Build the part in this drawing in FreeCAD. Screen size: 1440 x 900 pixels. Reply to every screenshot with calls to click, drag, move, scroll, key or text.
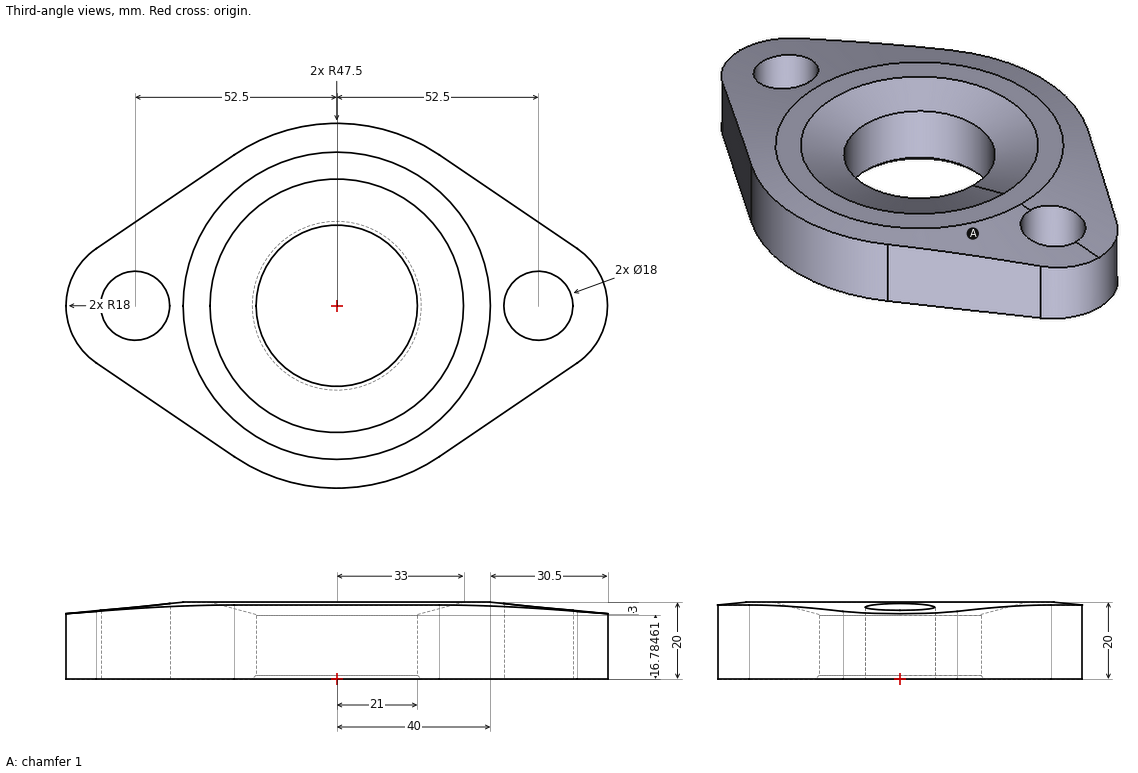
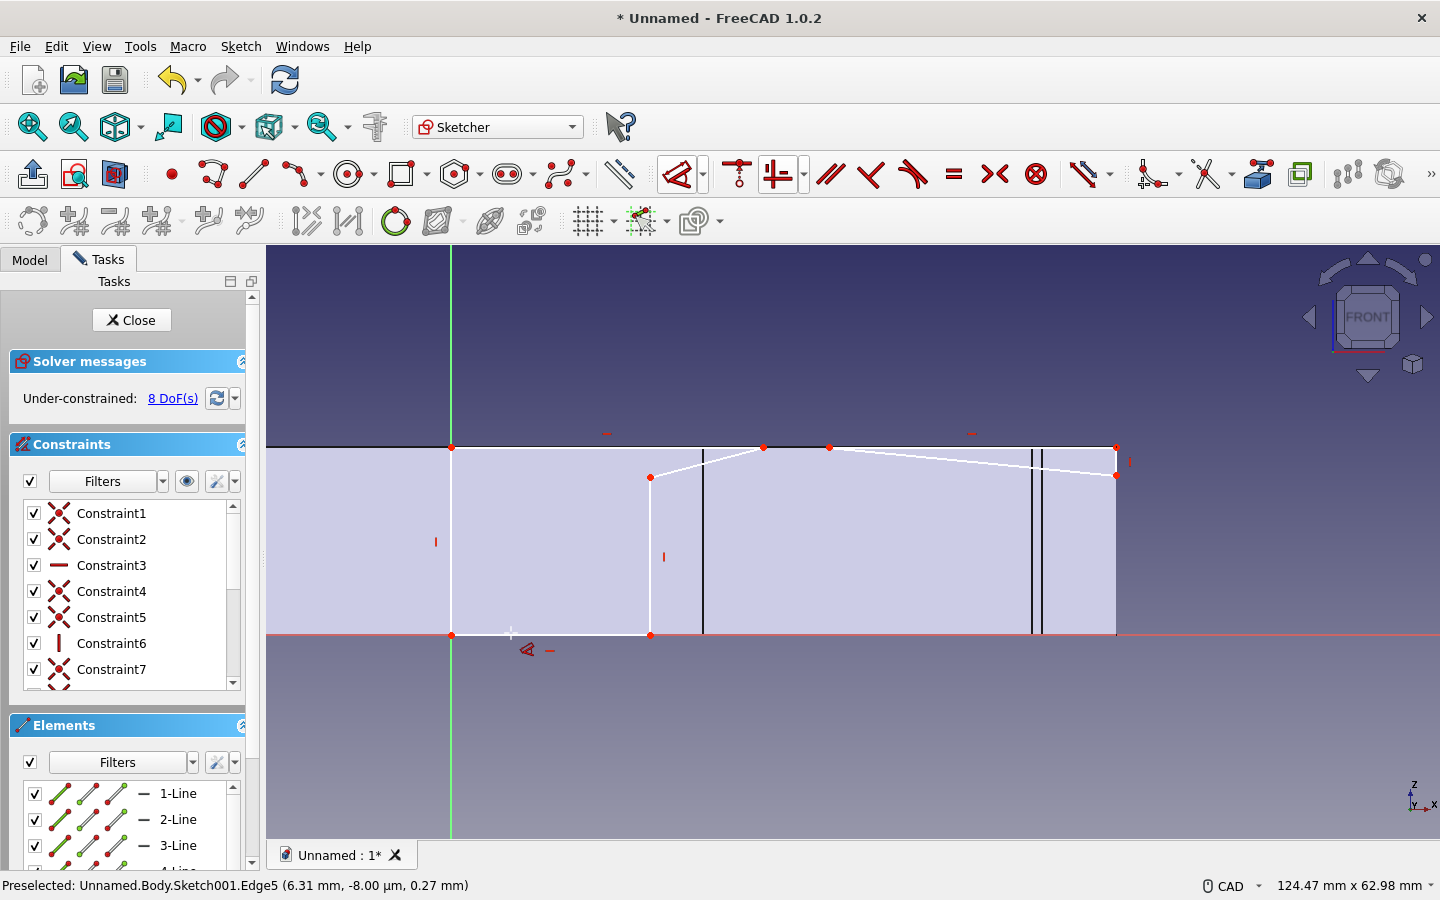
scroll(1116, 459, up, 2)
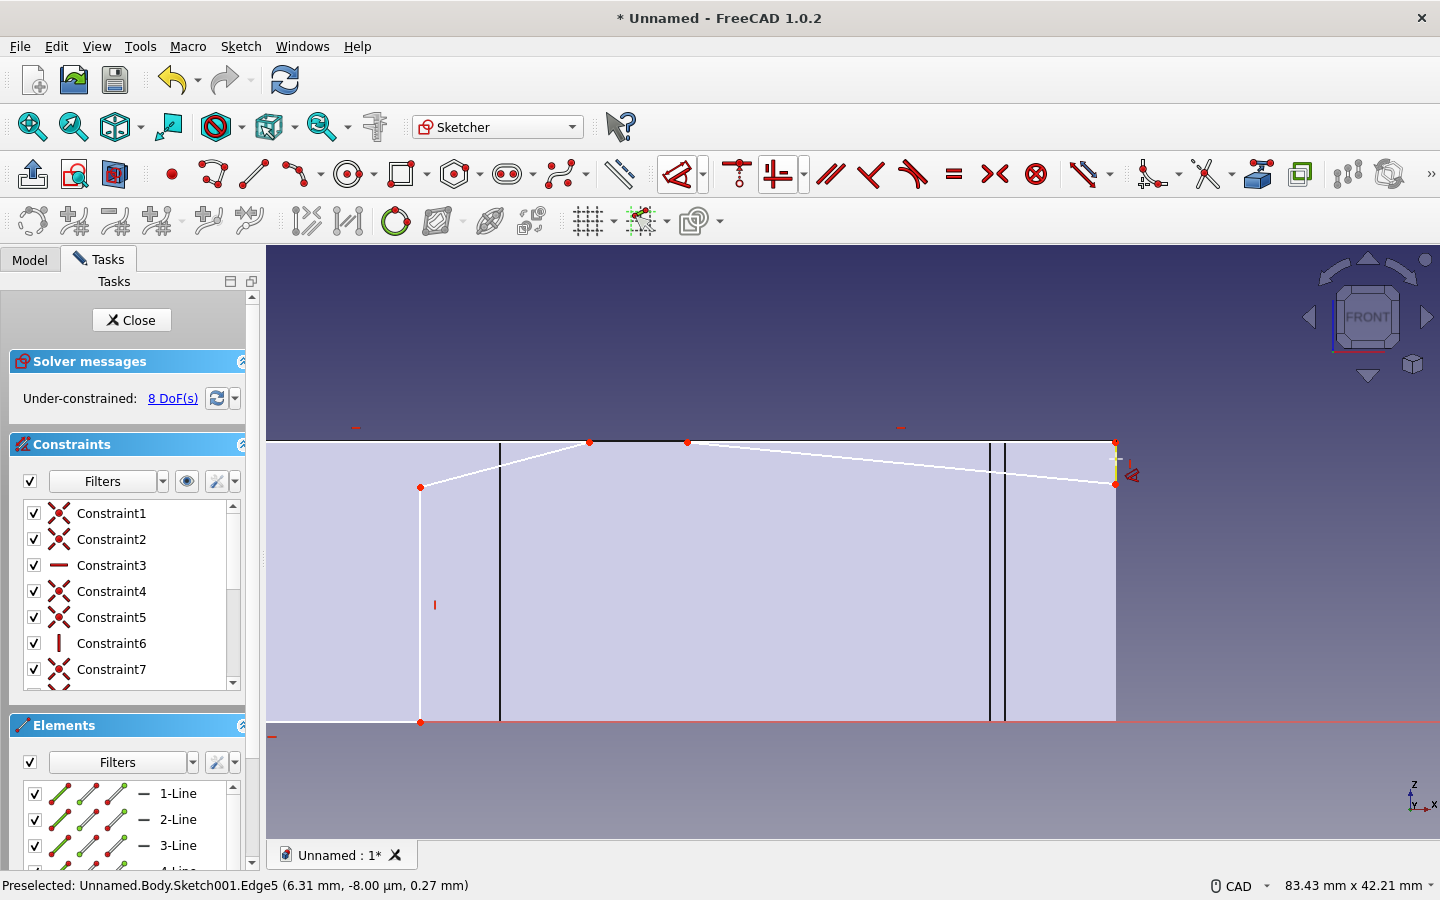
click(1116, 459)
click(1150, 463)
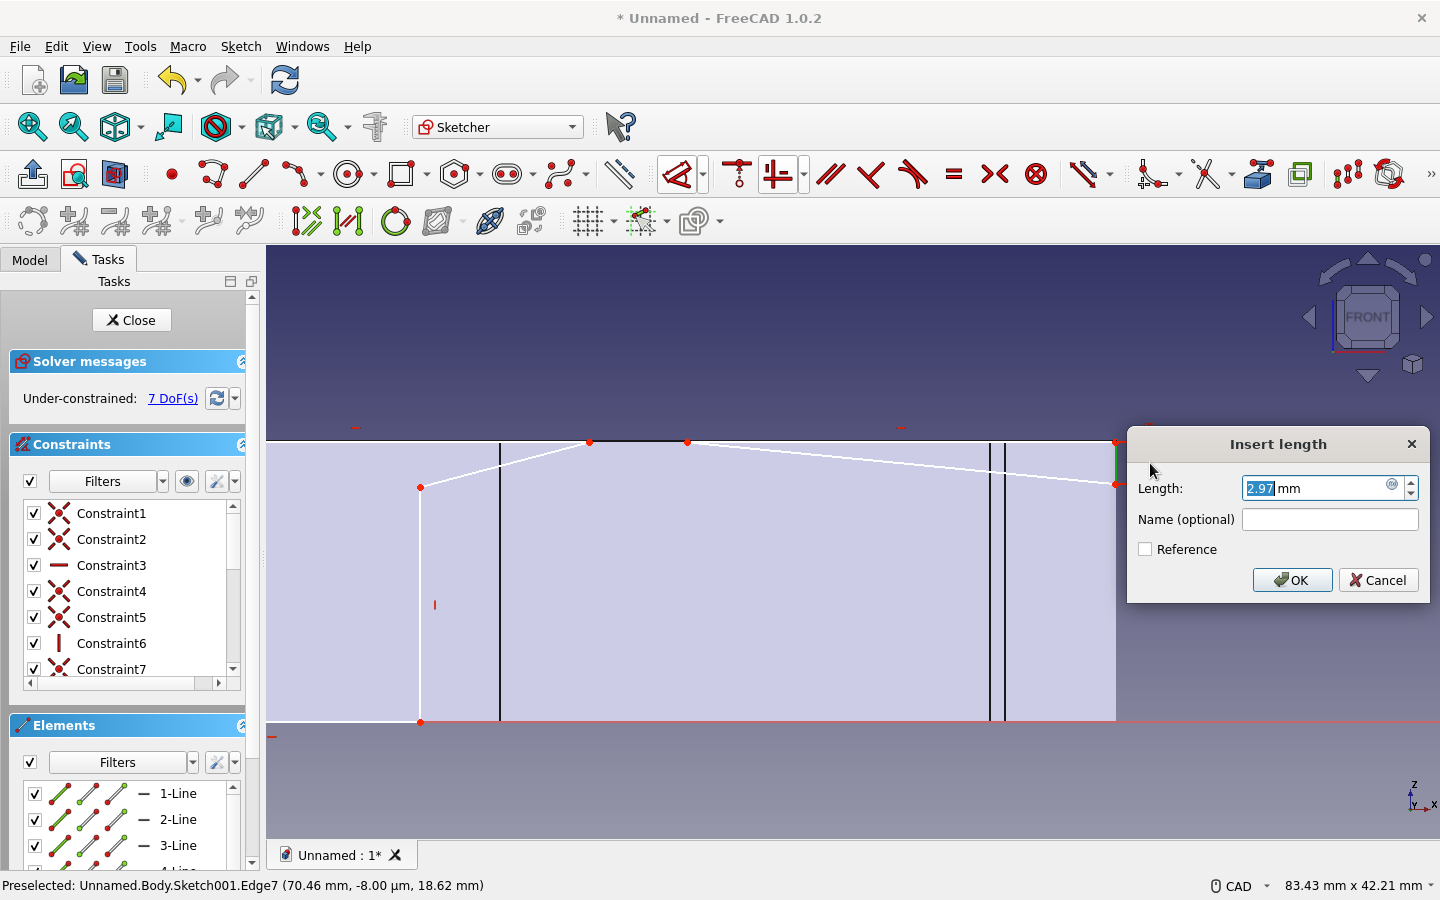
text(3)
key(Return)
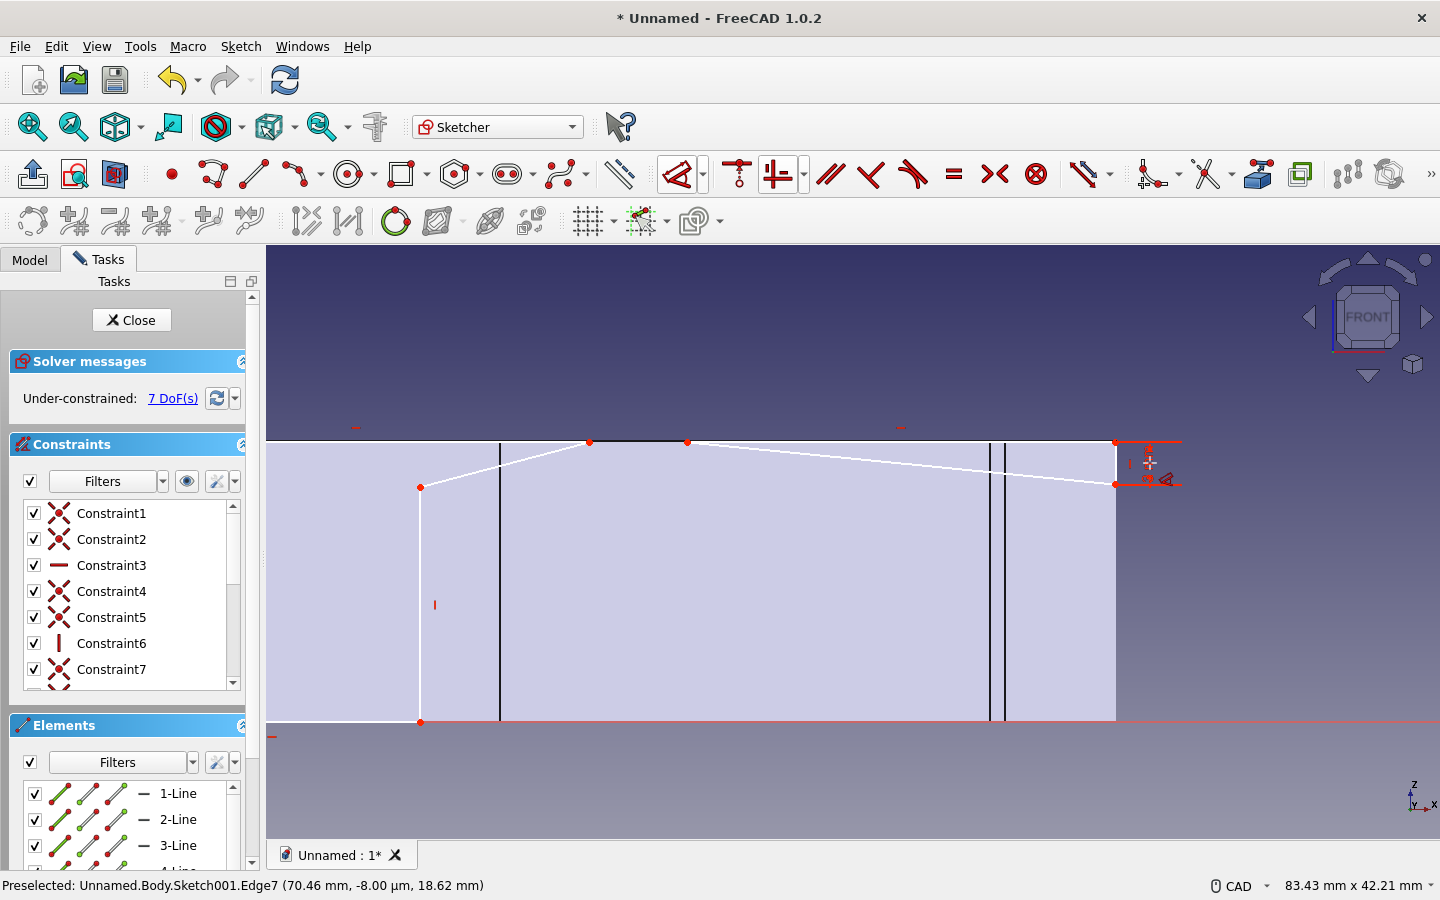
scroll(1118, 462, down, 2)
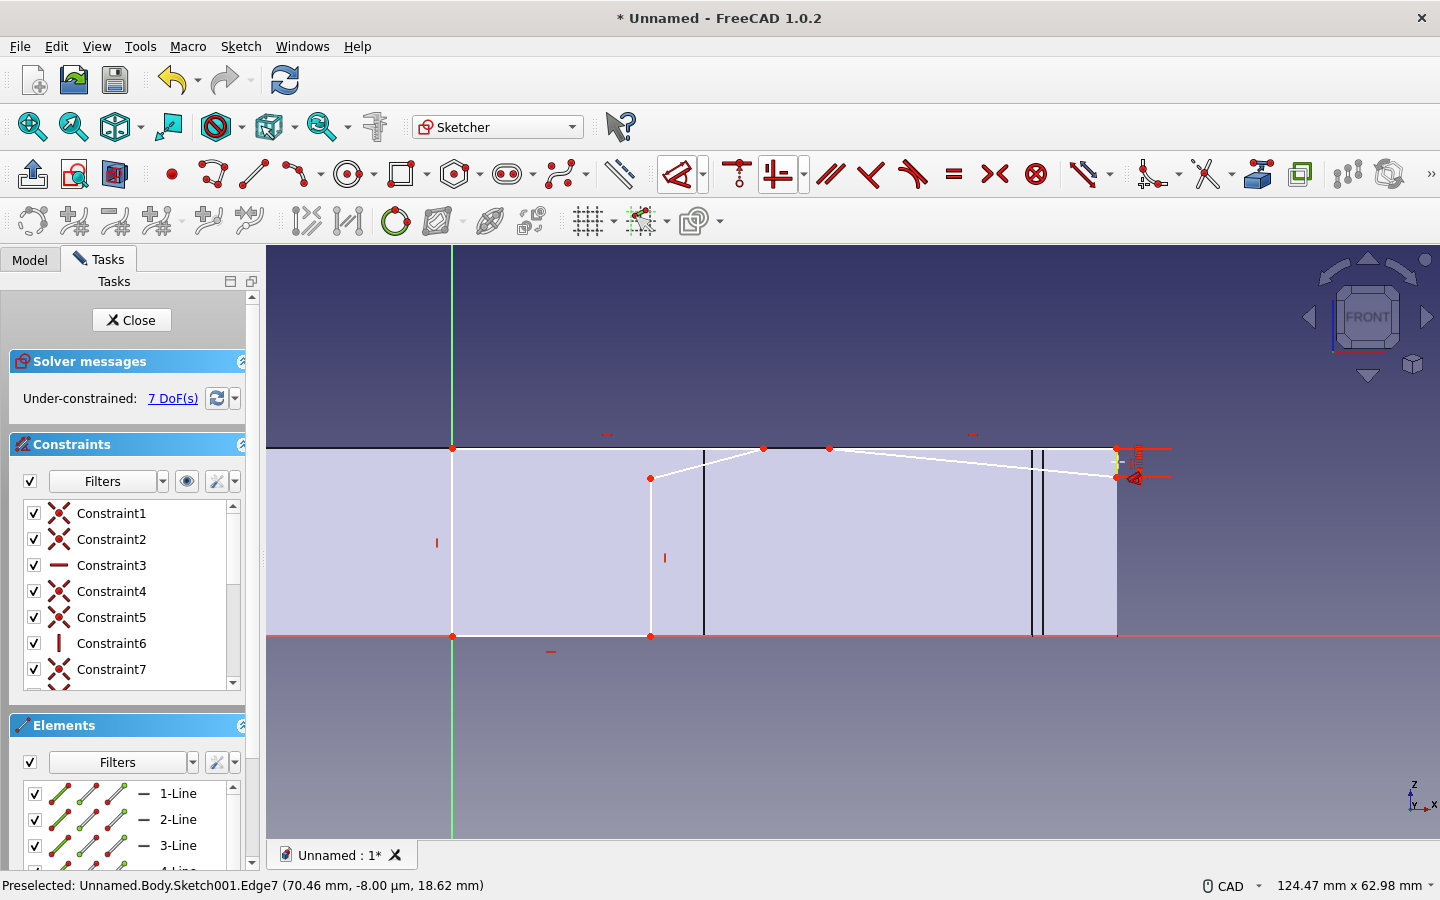
click(452, 580)
click(418, 543)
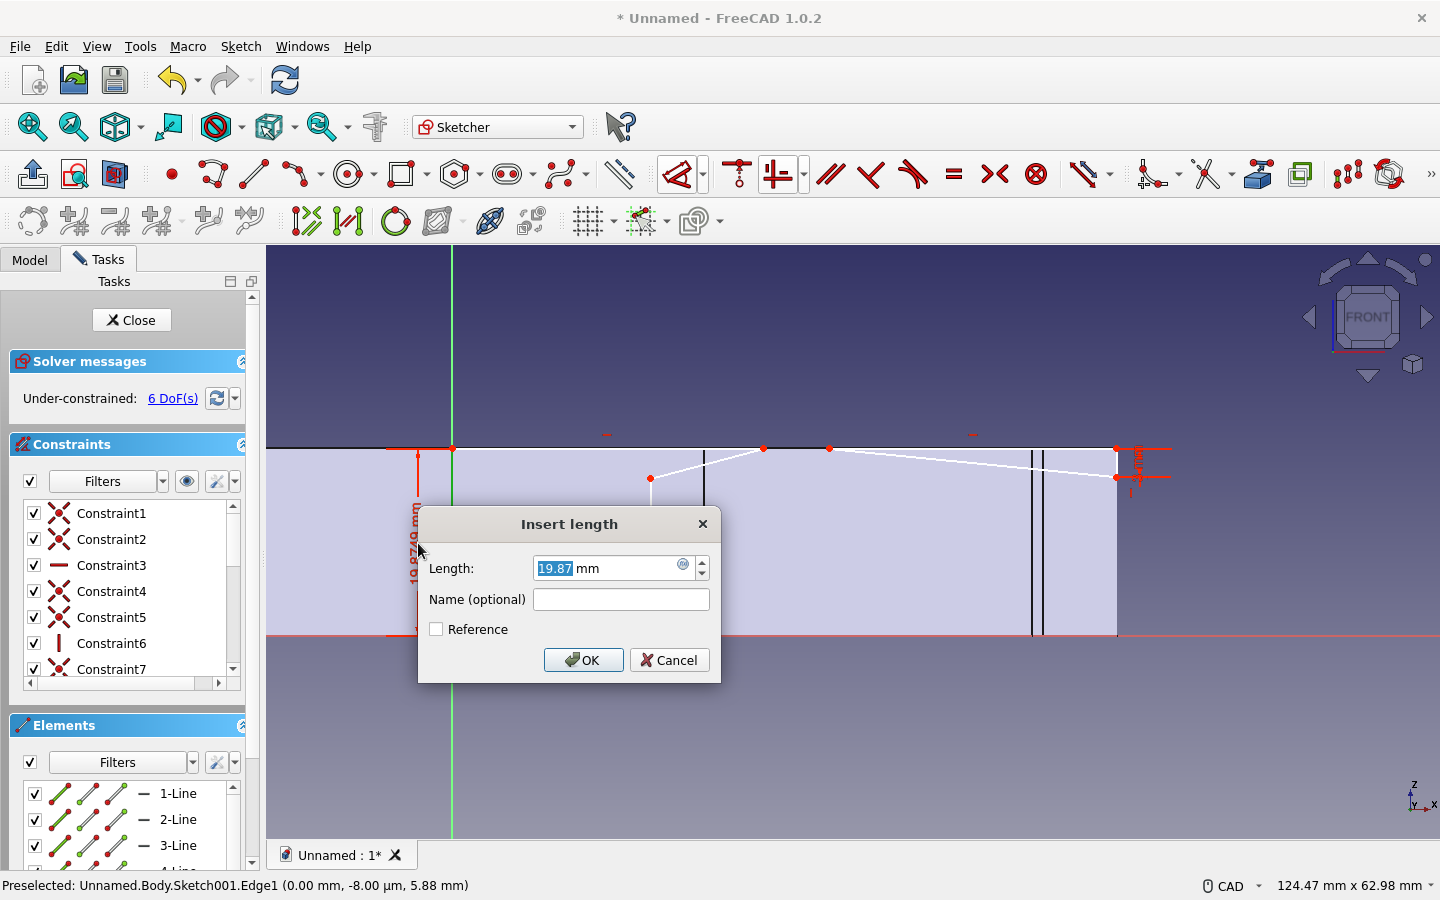
text(20)
key(Return)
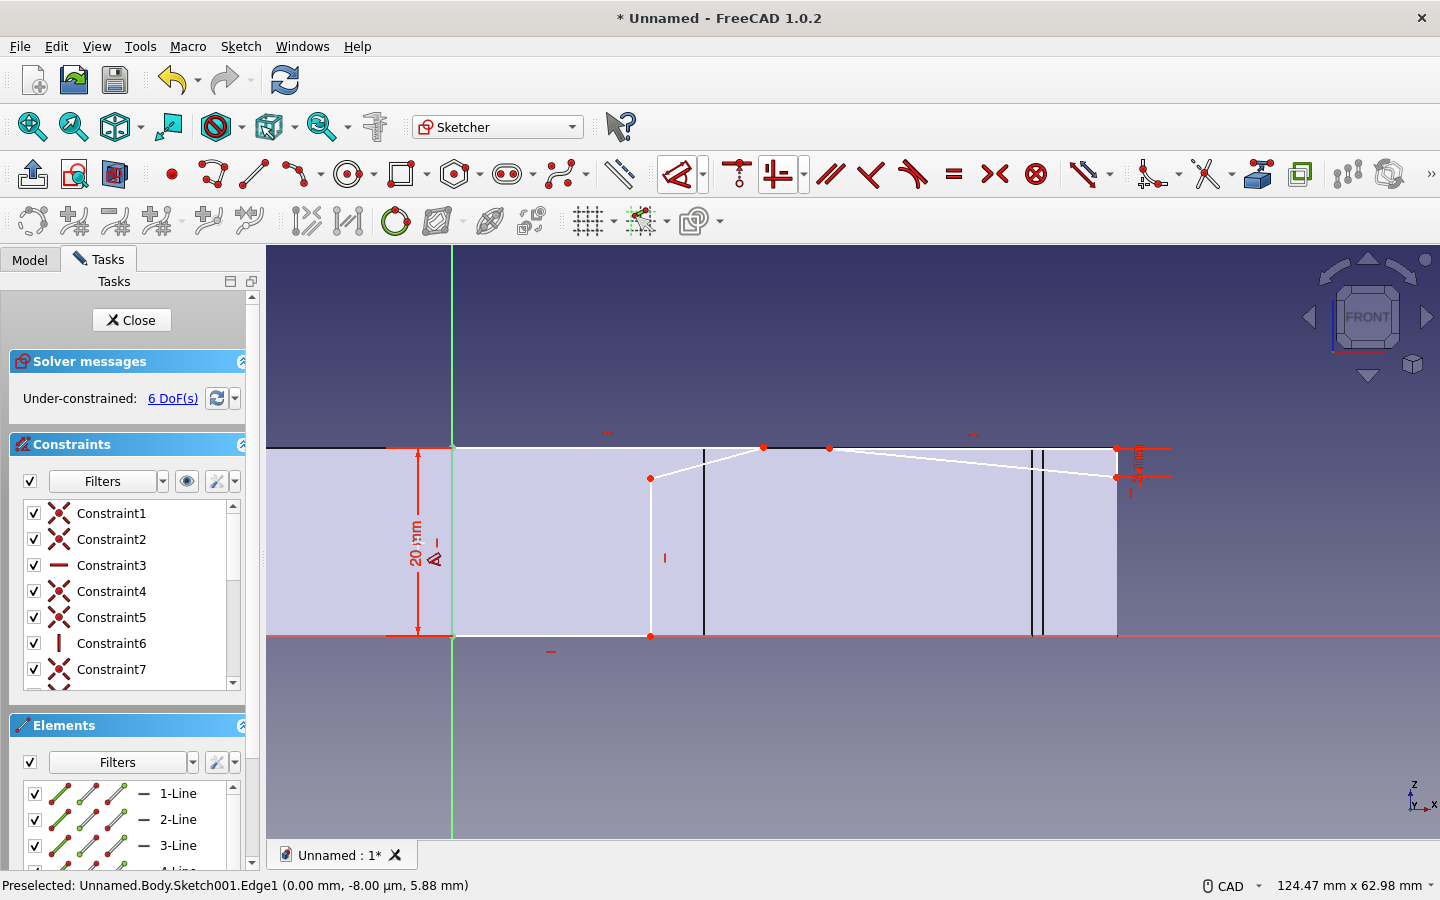
click(546, 448)
click(608, 414)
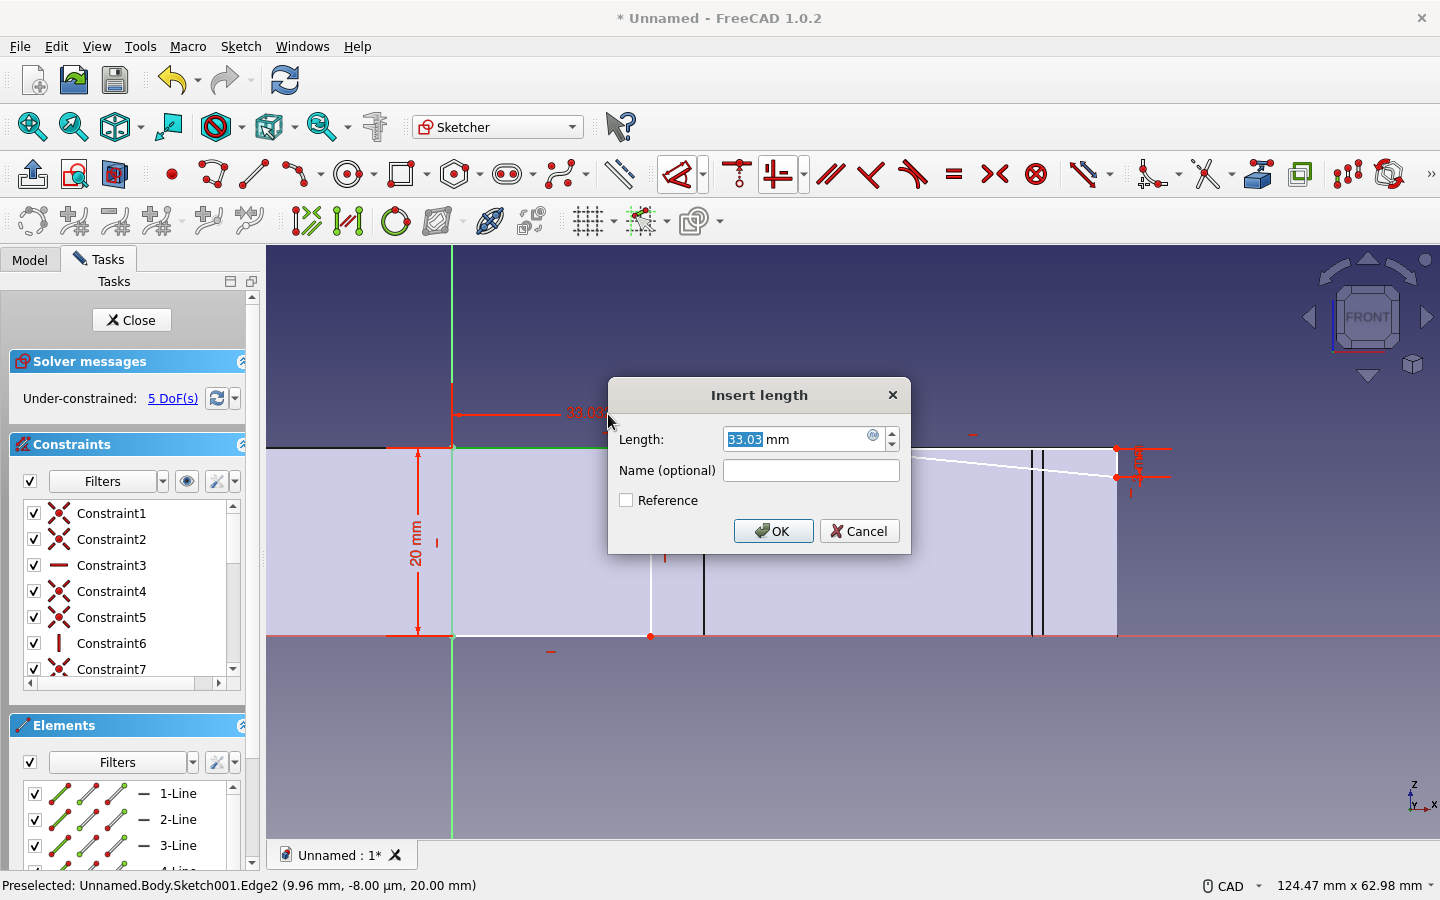
text(33)
key(Return)